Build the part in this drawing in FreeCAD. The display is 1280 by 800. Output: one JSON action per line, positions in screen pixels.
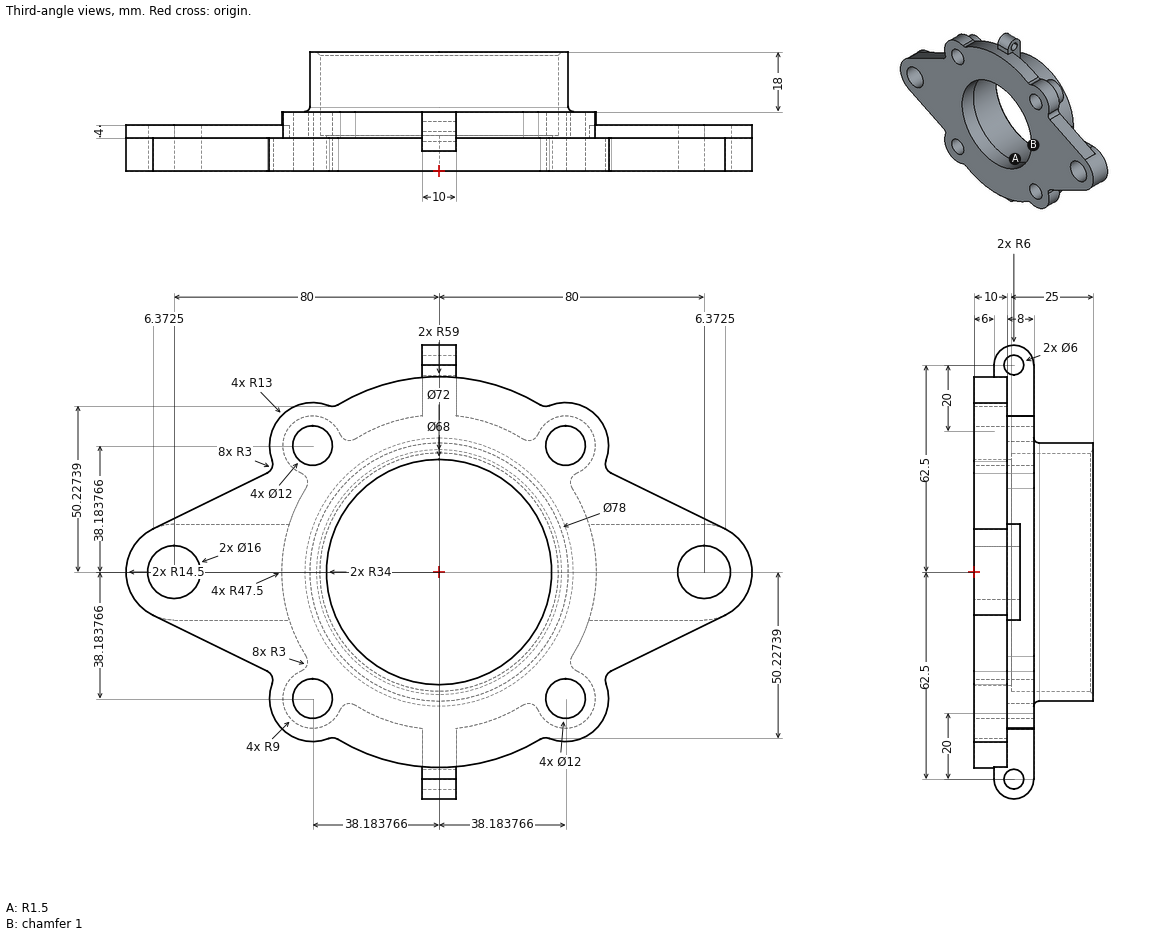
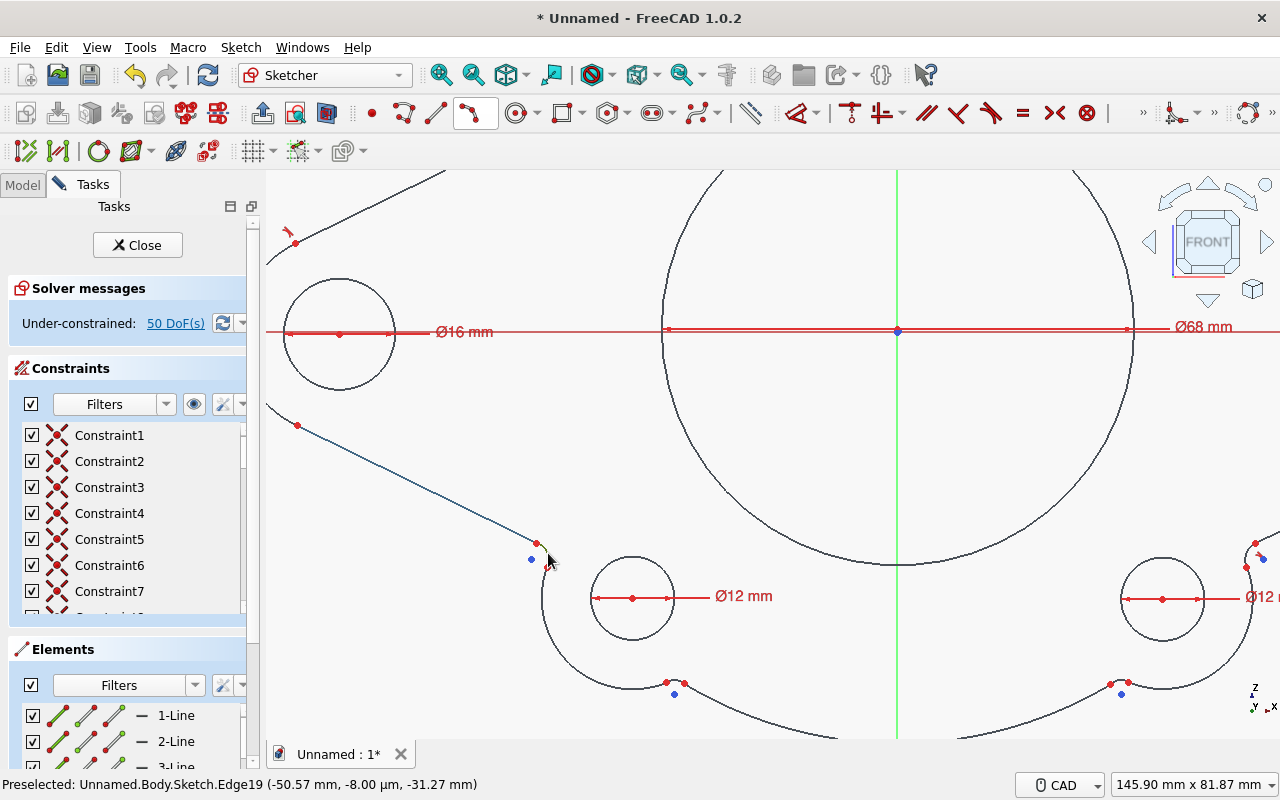
{"action": "left_click", "coordinate": [992, 114]}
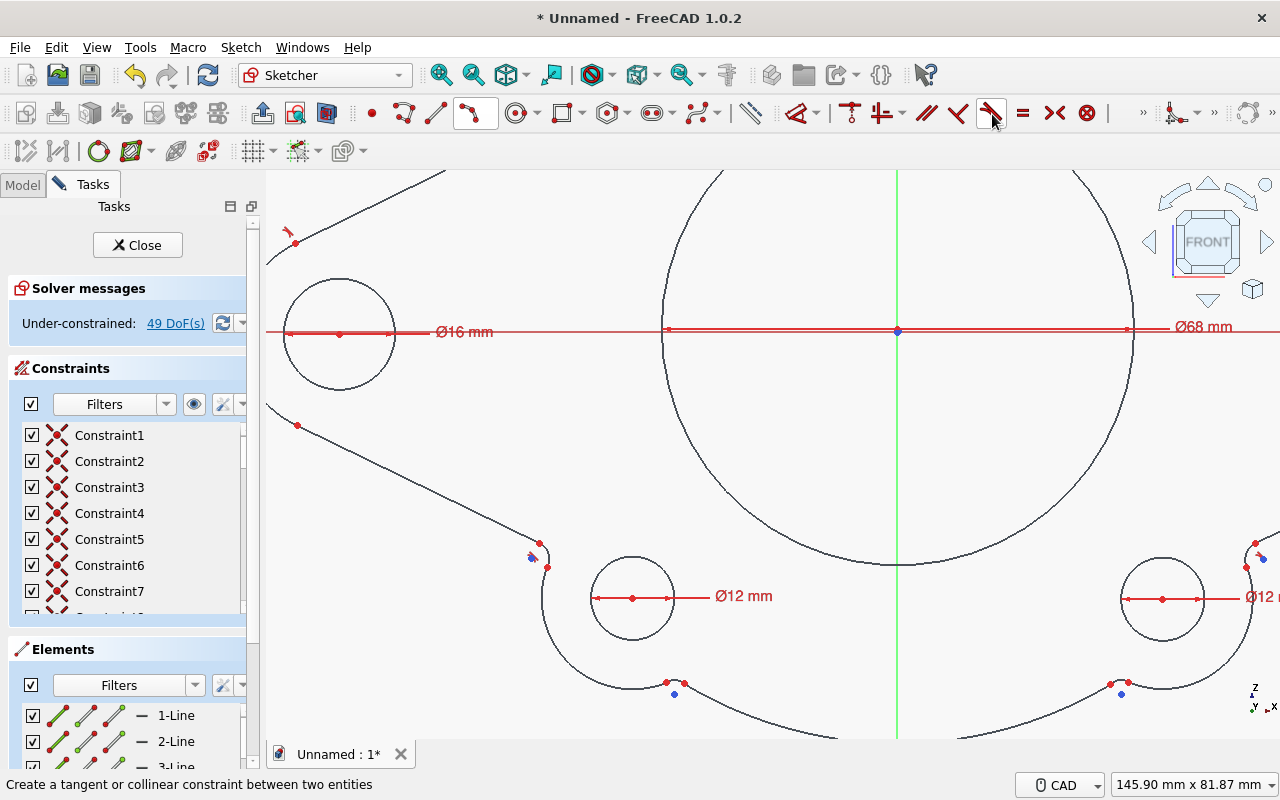
{"action": "left_click", "coordinate": [467, 508]}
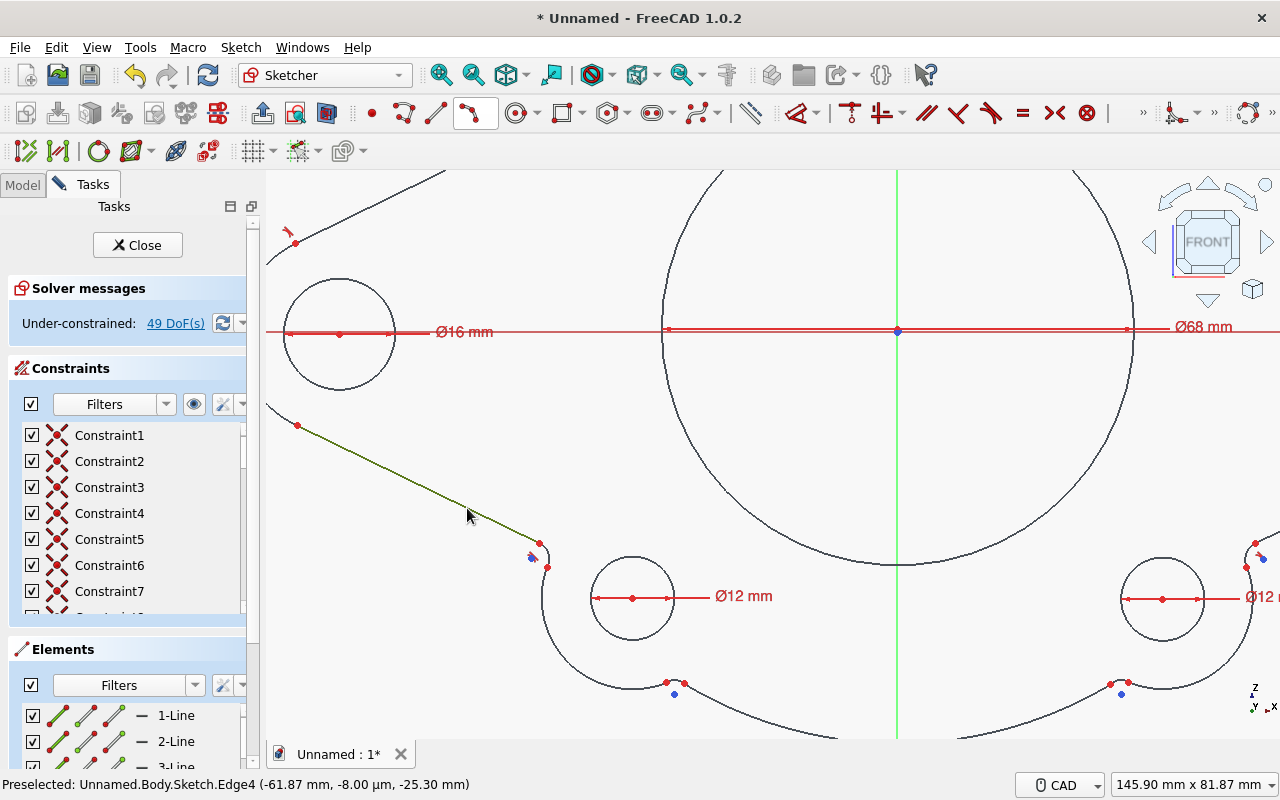
{"action": "scroll", "coordinate": [547, 554], "scroll_direction": "down", "scroll_amount": 4}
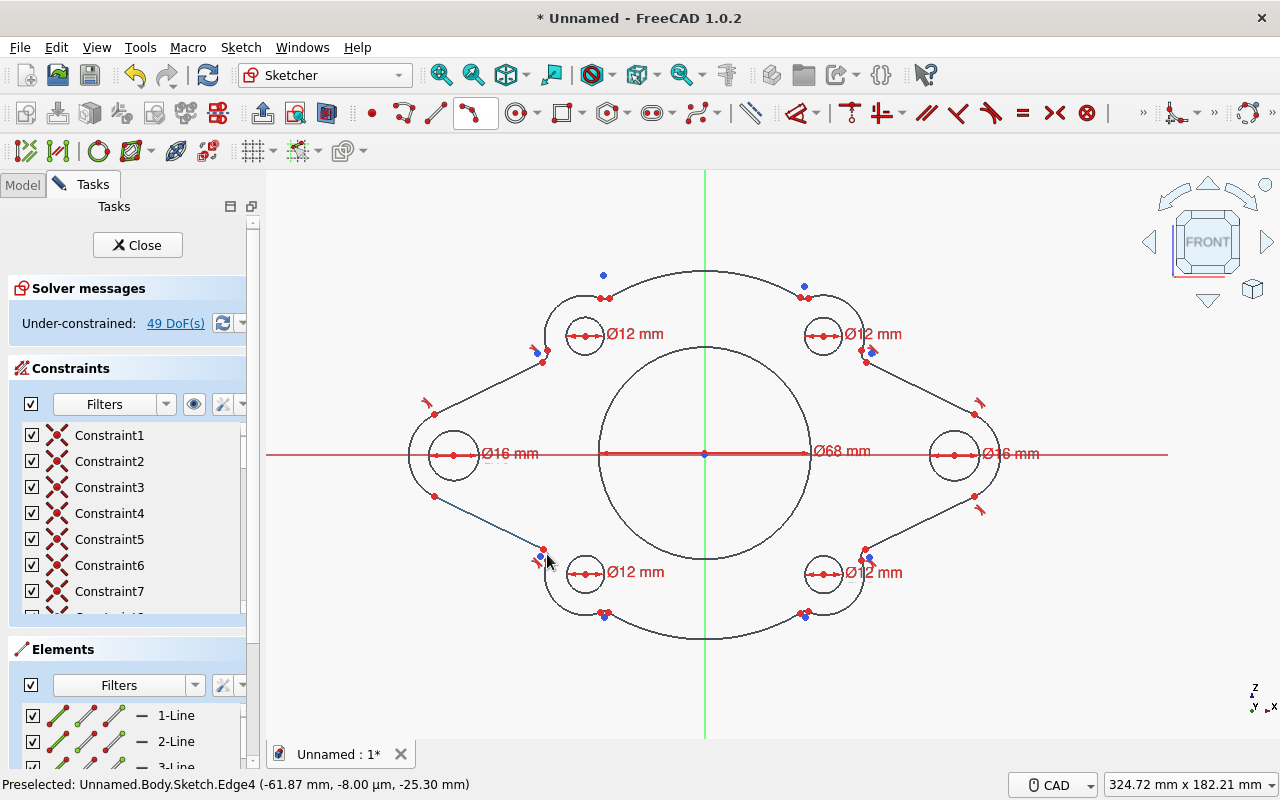
{"action": "left_click", "coordinate": [413, 436]}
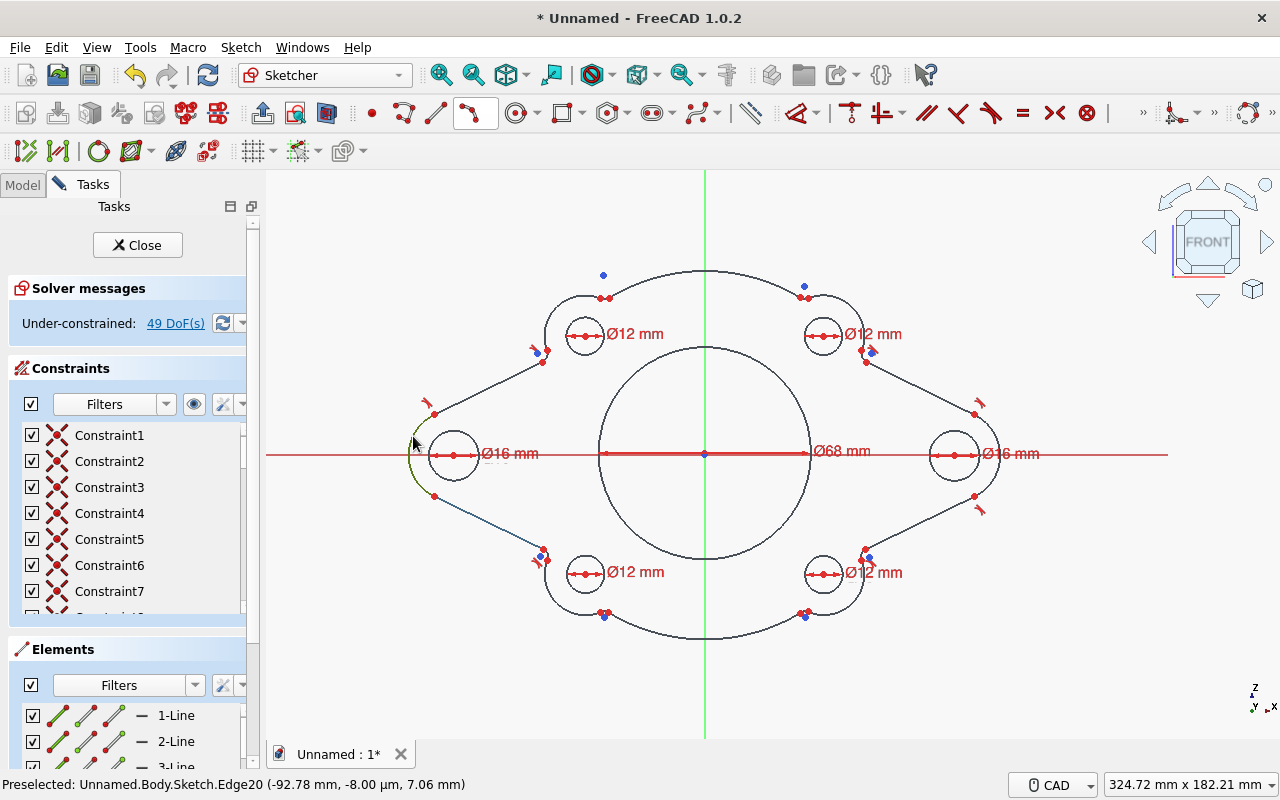
{"action": "left_click", "coordinate": [992, 114]}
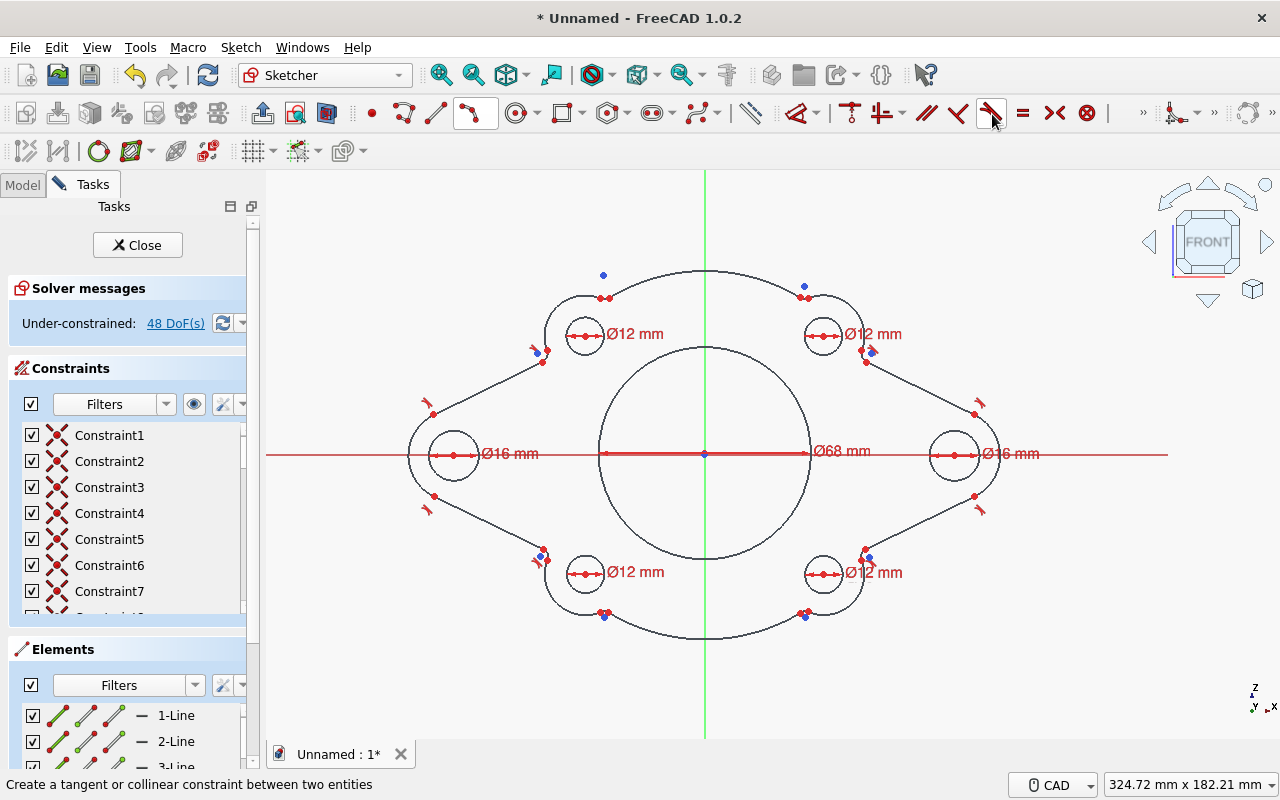
{"action": "scroll", "coordinate": [547, 357], "scroll_direction": "up", "scroll_amount": 4}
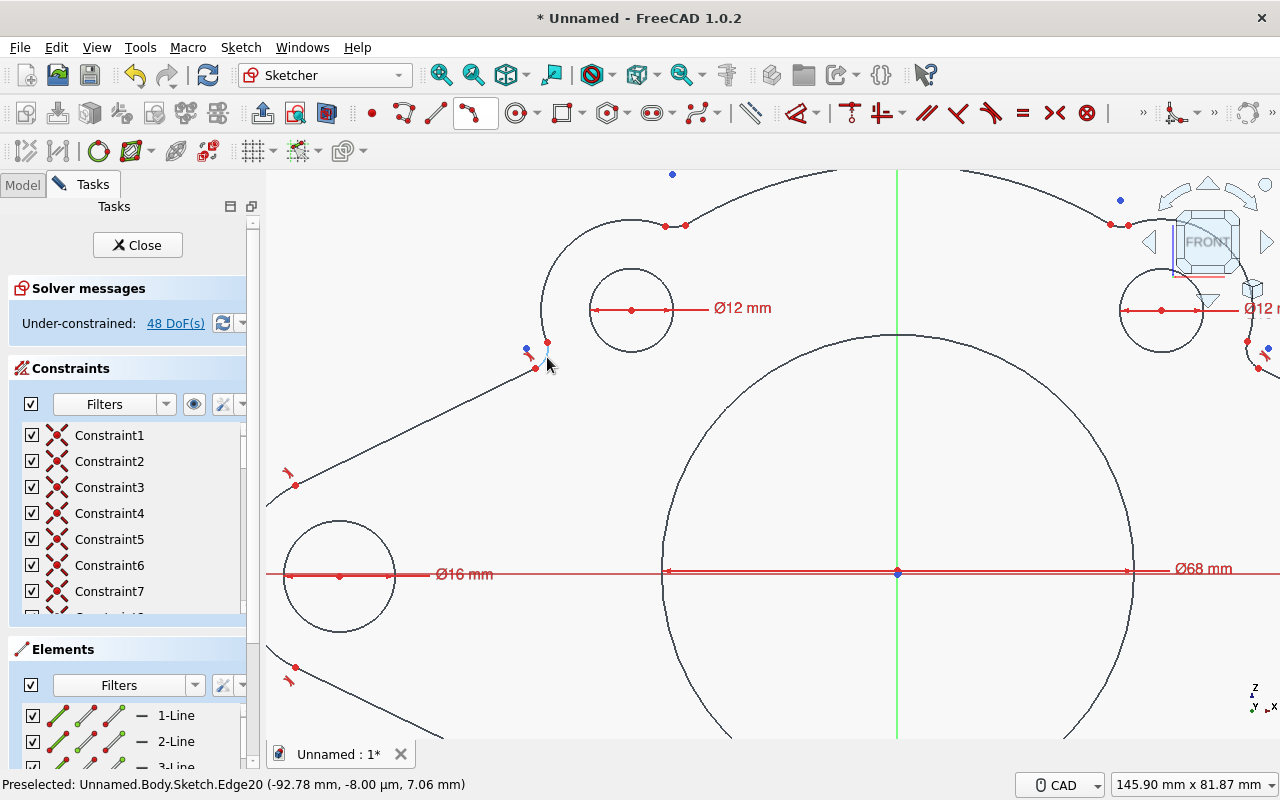
{"action": "left_click", "coordinate": [546, 357]}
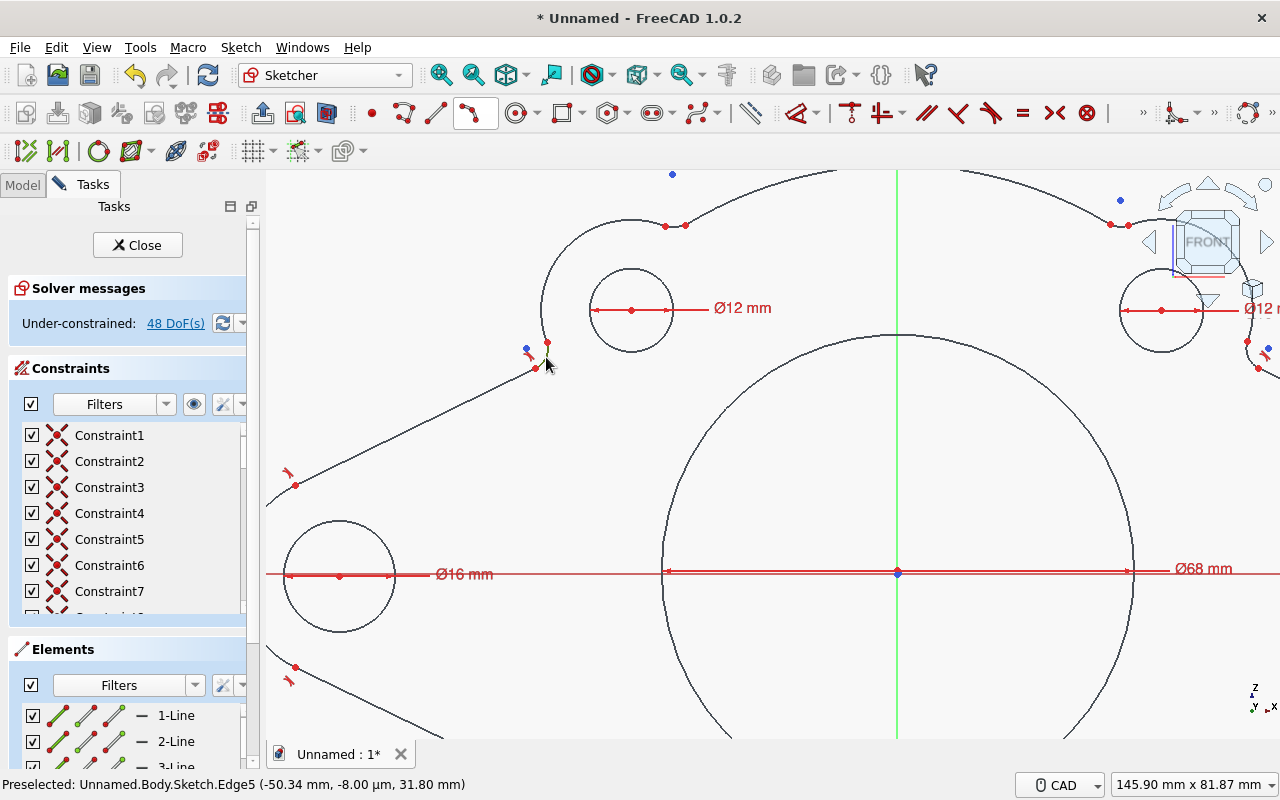
{"action": "left_click", "coordinate": [604, 224]}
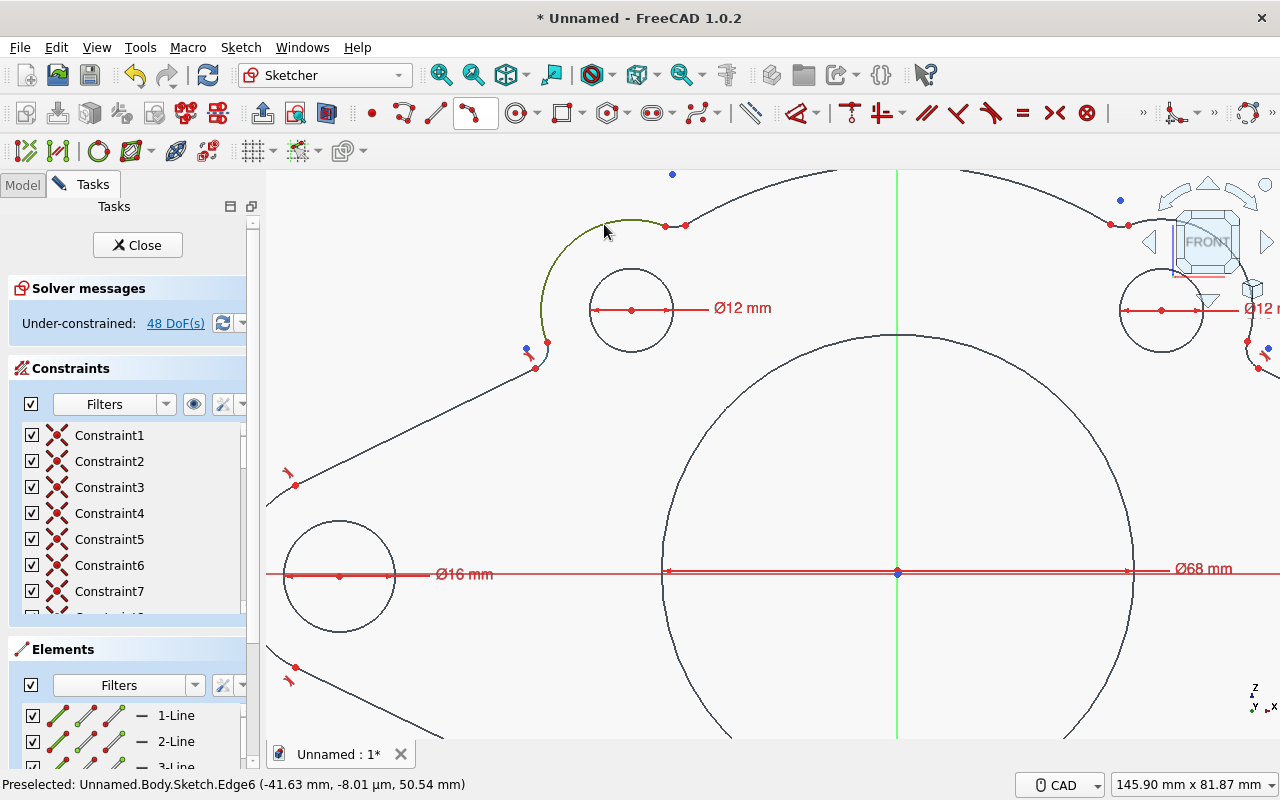
{"action": "left_click", "coordinate": [992, 114]}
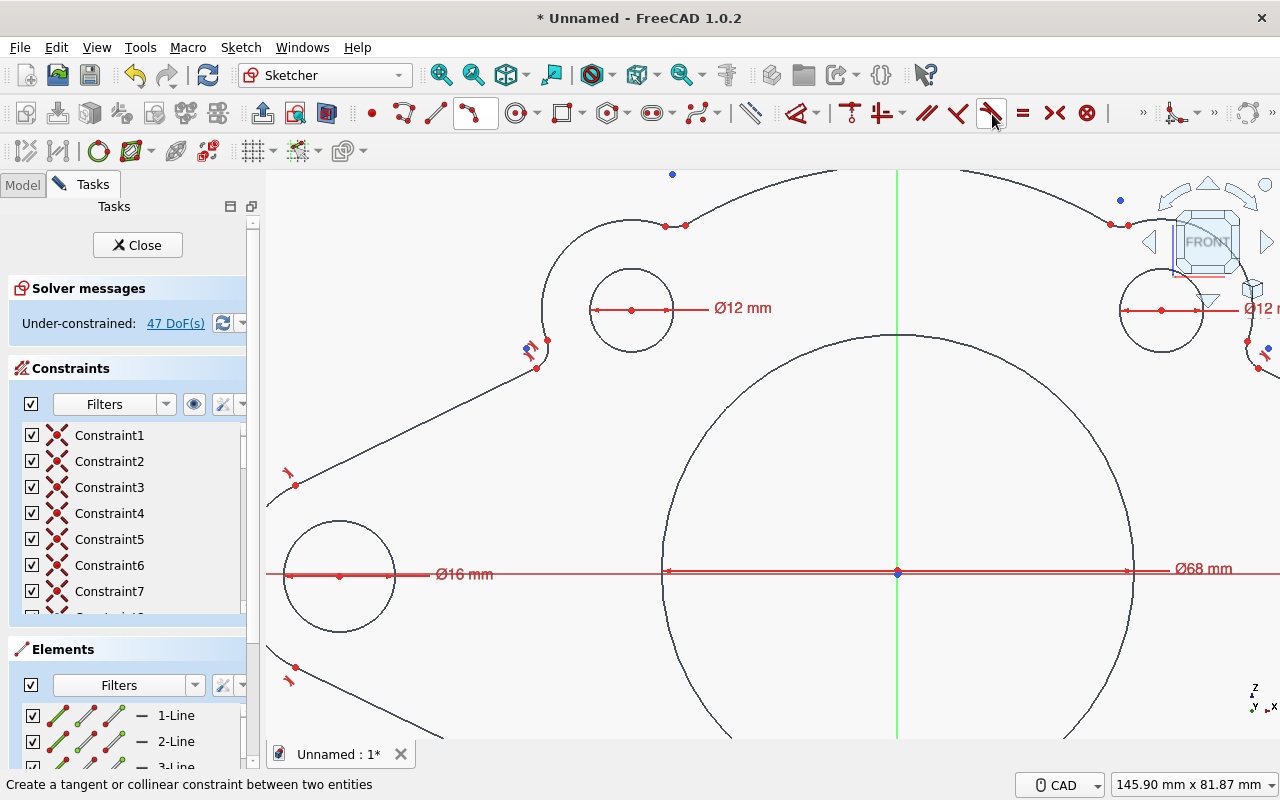
{"action": "left_click", "coordinate": [605, 224]}